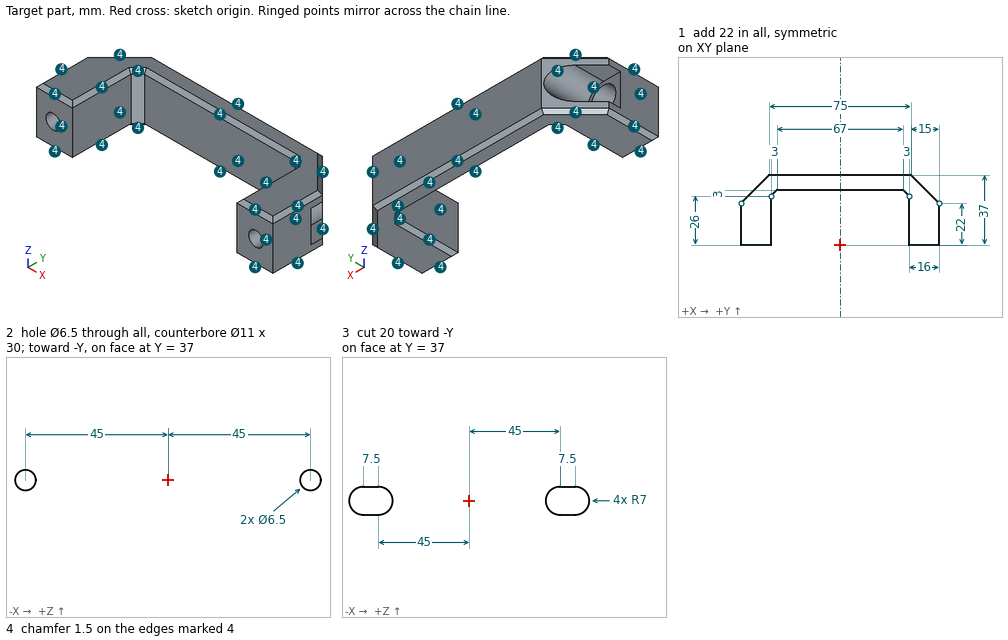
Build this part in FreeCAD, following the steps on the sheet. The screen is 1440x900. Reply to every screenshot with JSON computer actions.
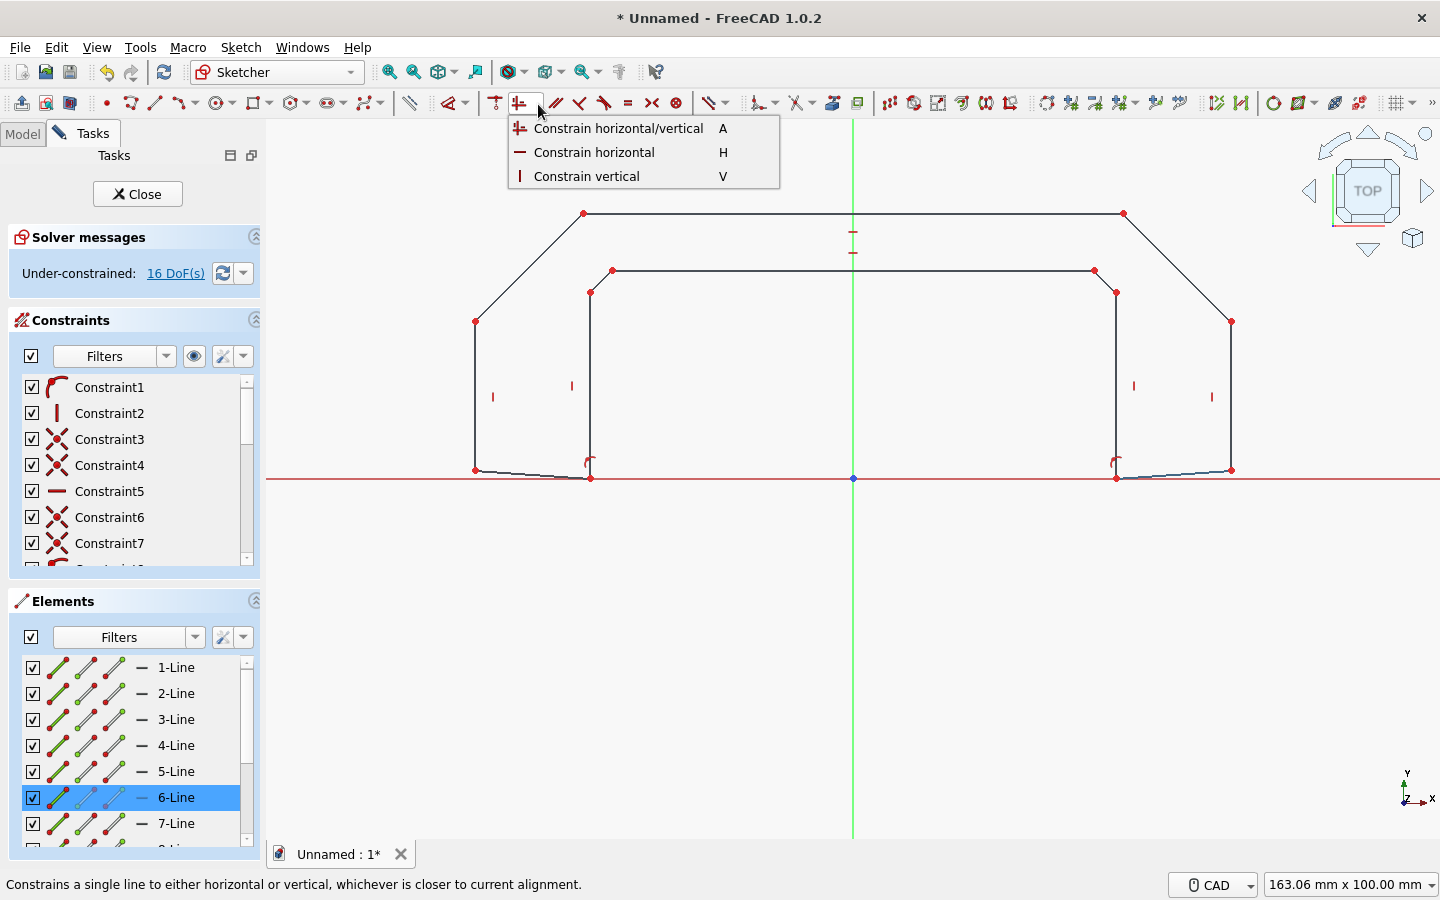
{"action": "left_click", "coordinate": [644, 152]}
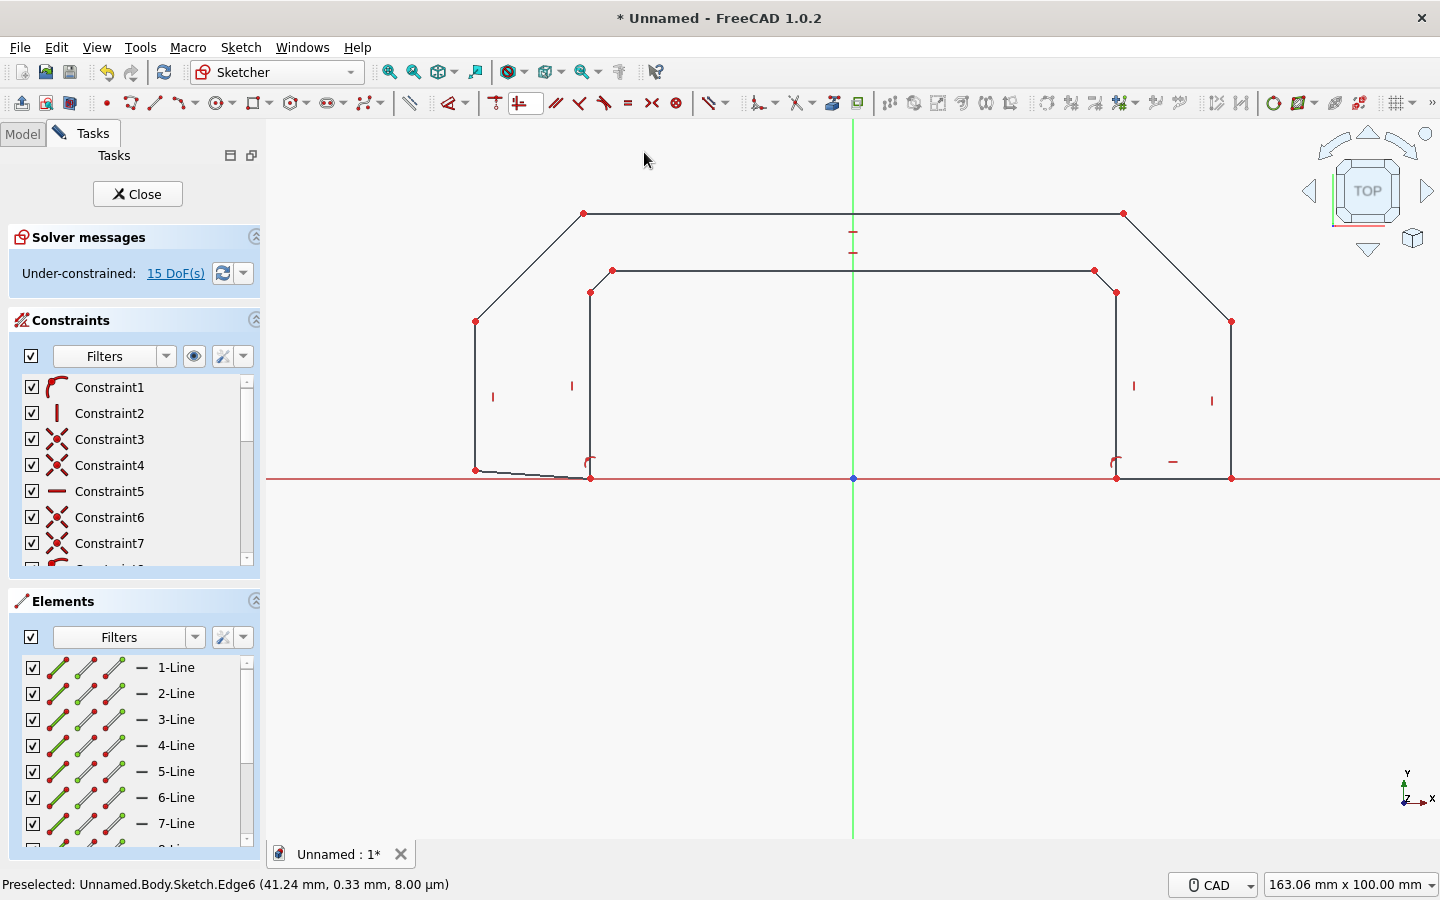
{"action": "left_click", "coordinate": [556, 477]}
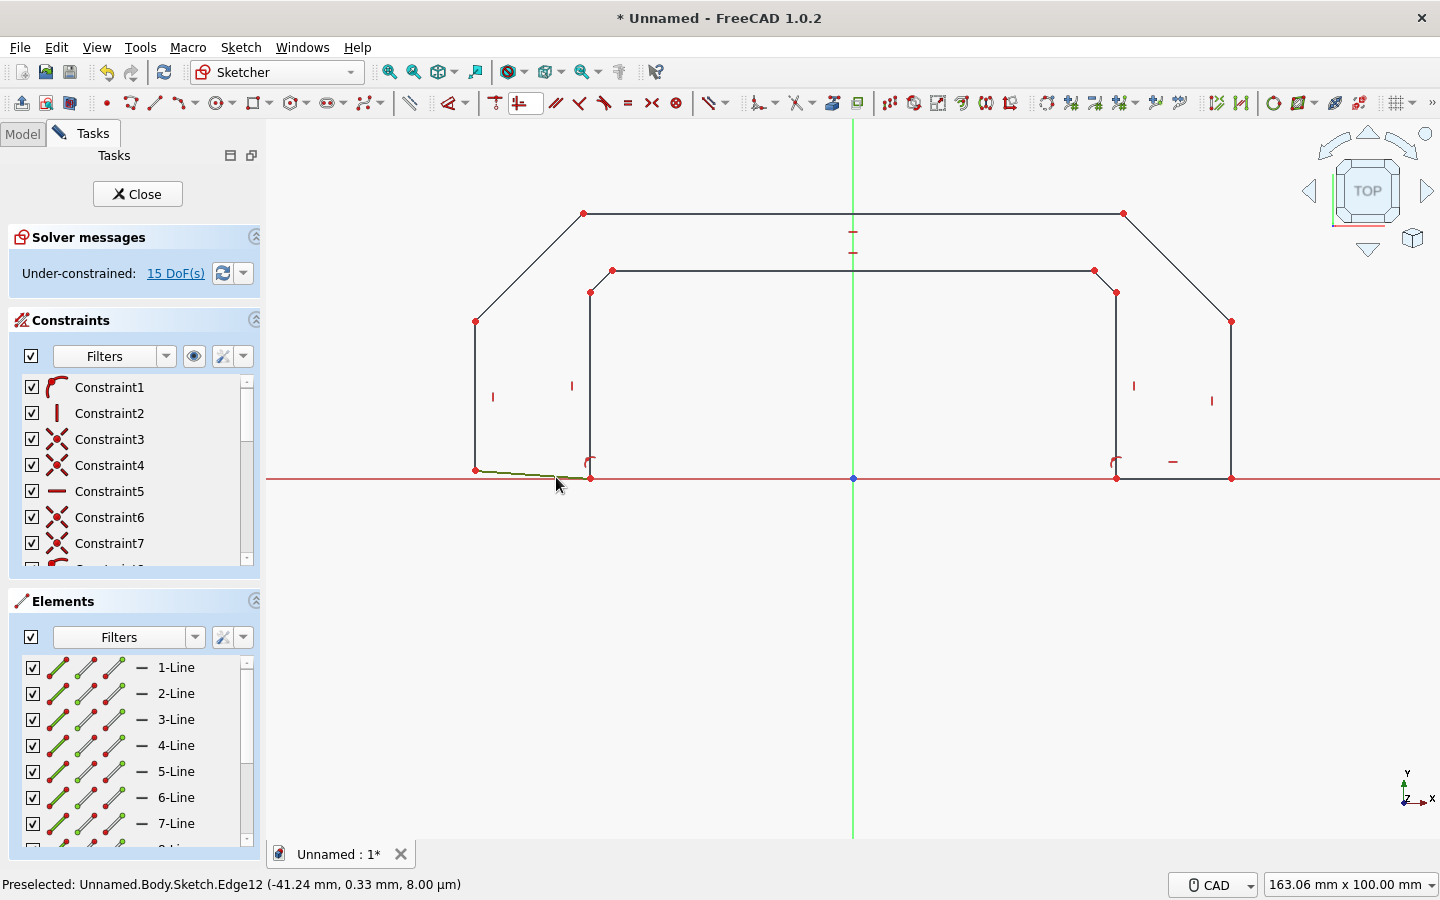
{"action": "key", "text": "h"}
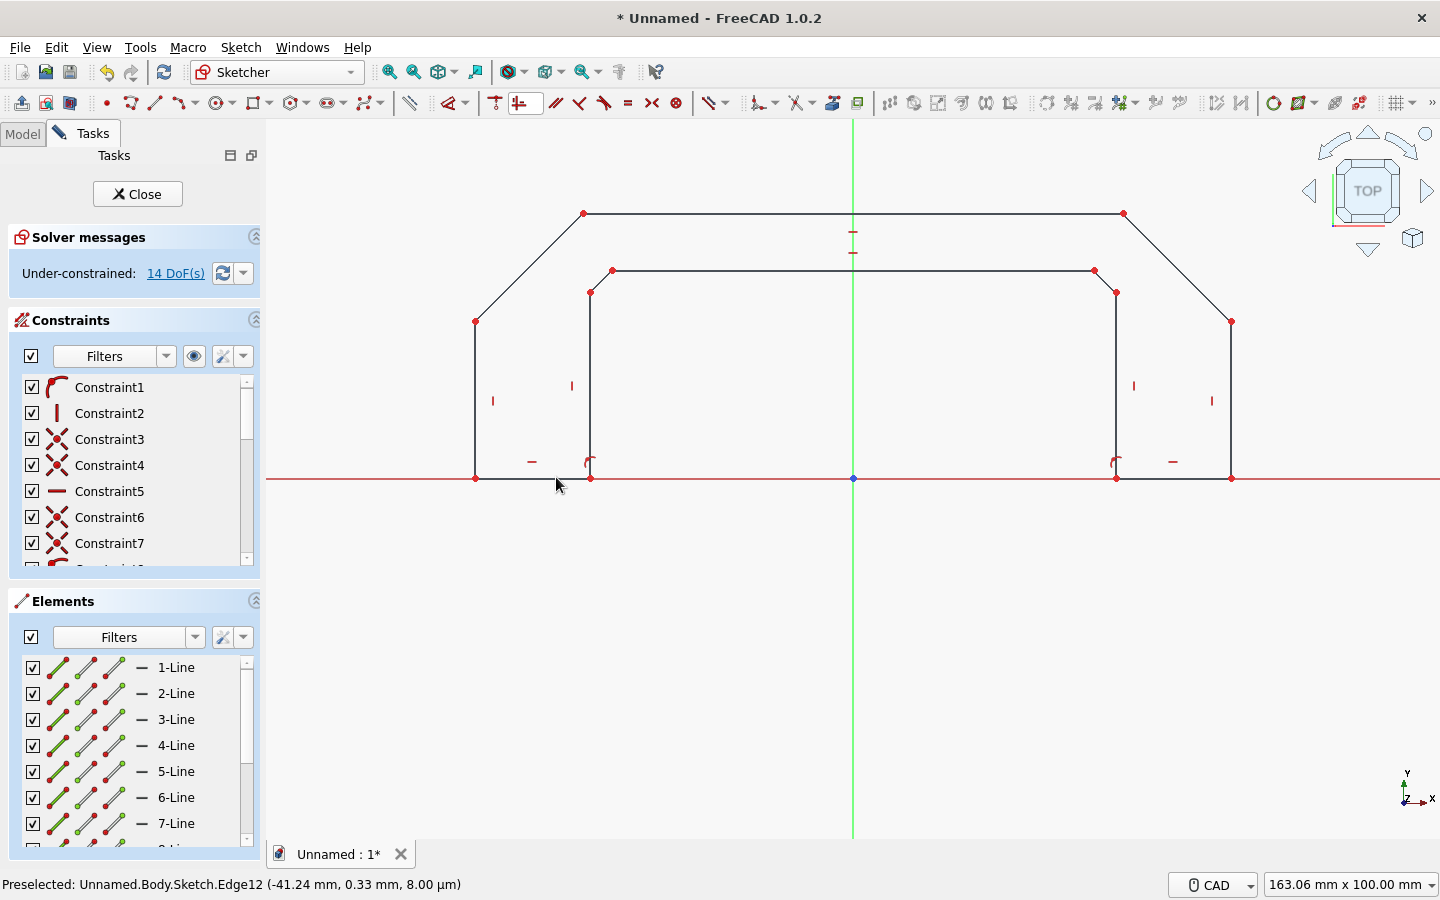
{"action": "left_click", "coordinate": [590, 293]}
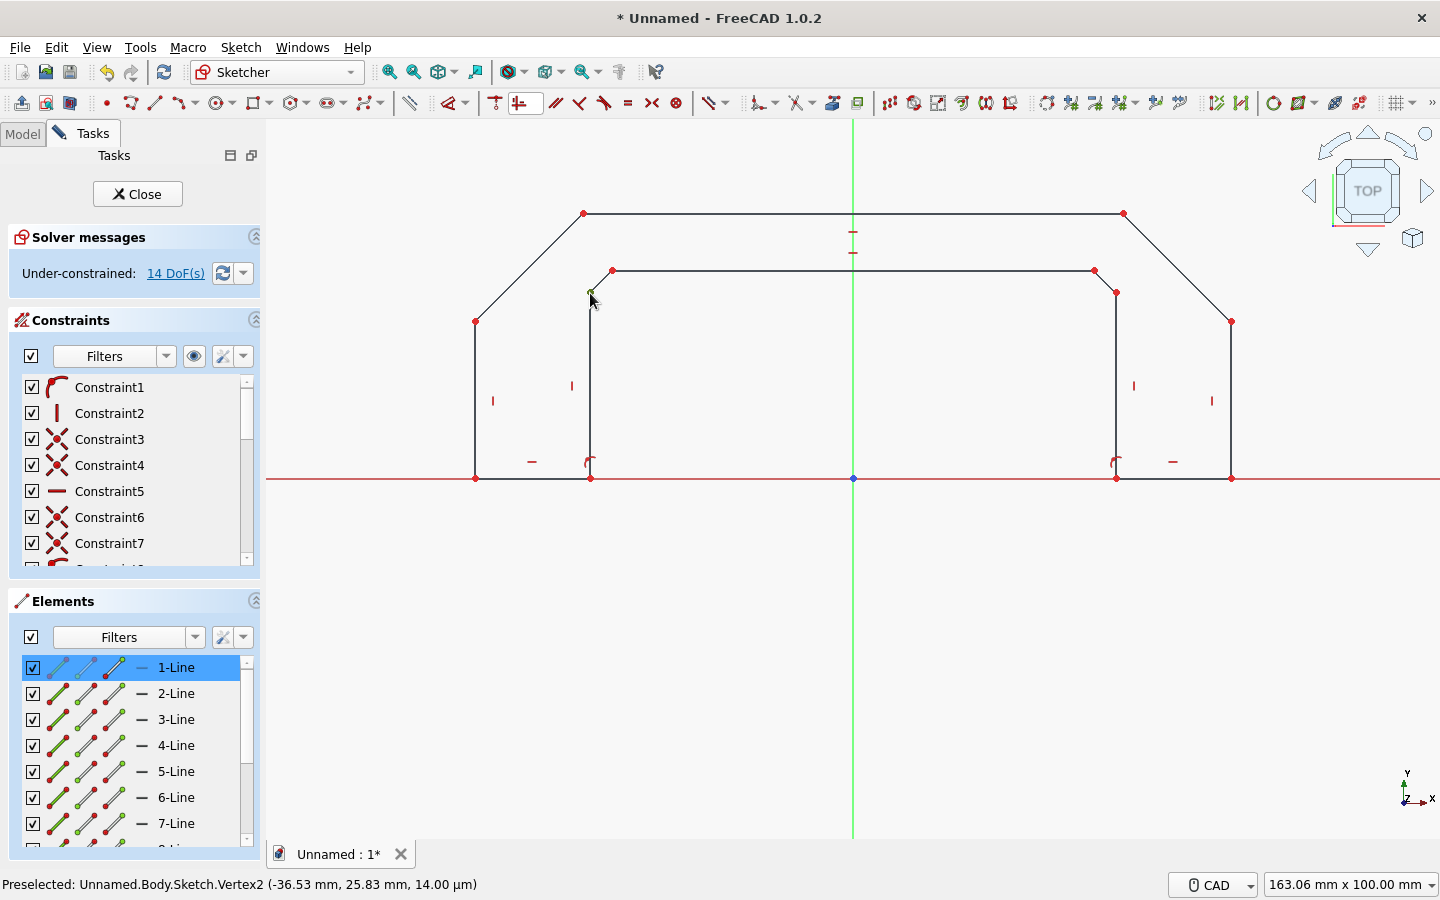
{"action": "left_click", "coordinate": [1116, 293]}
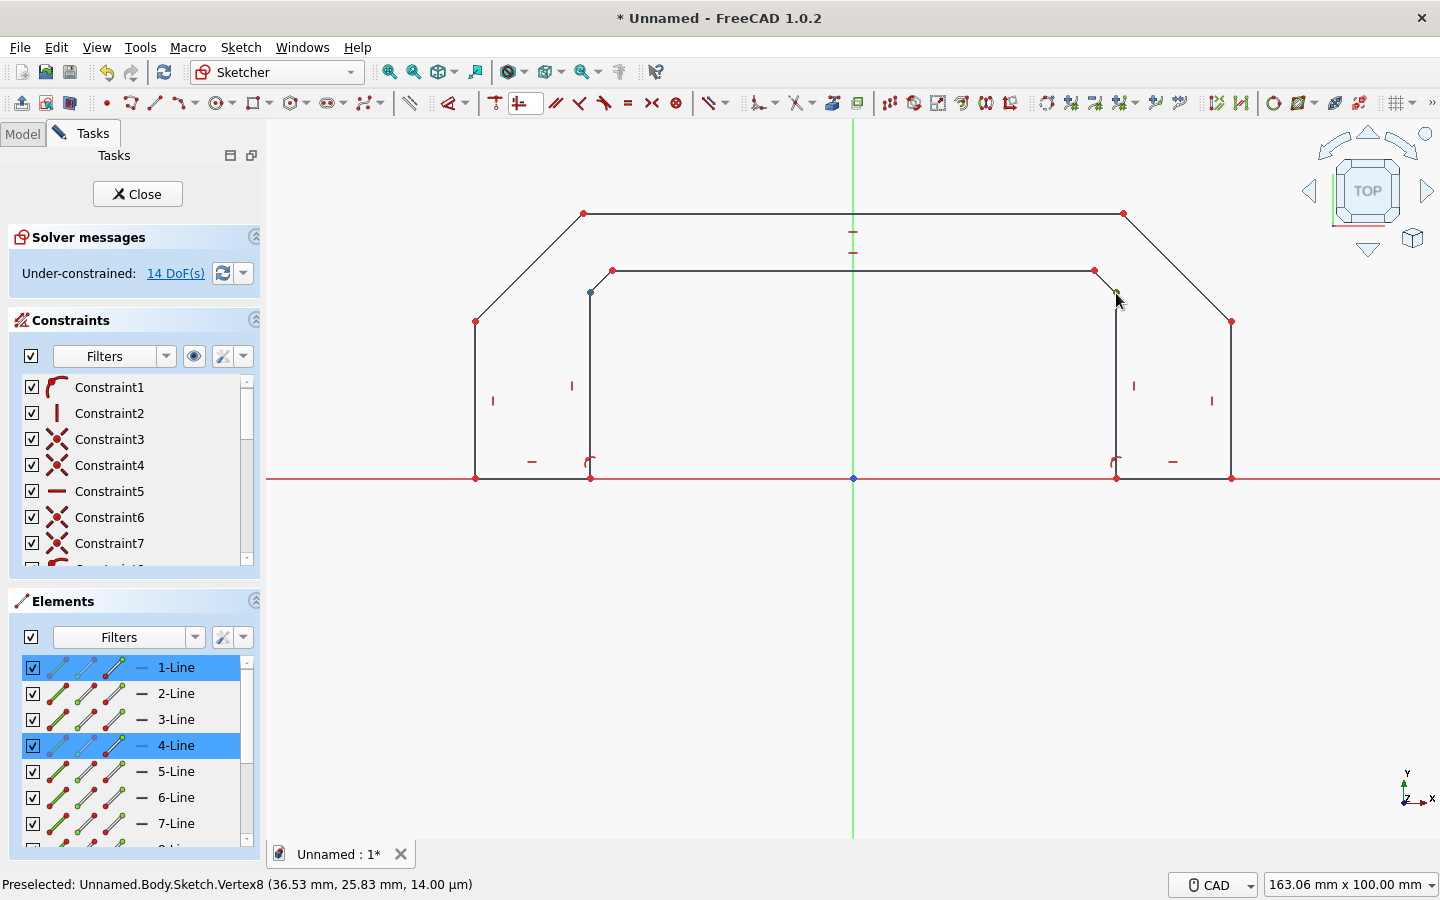
{"action": "left_click", "coordinate": [853, 764]}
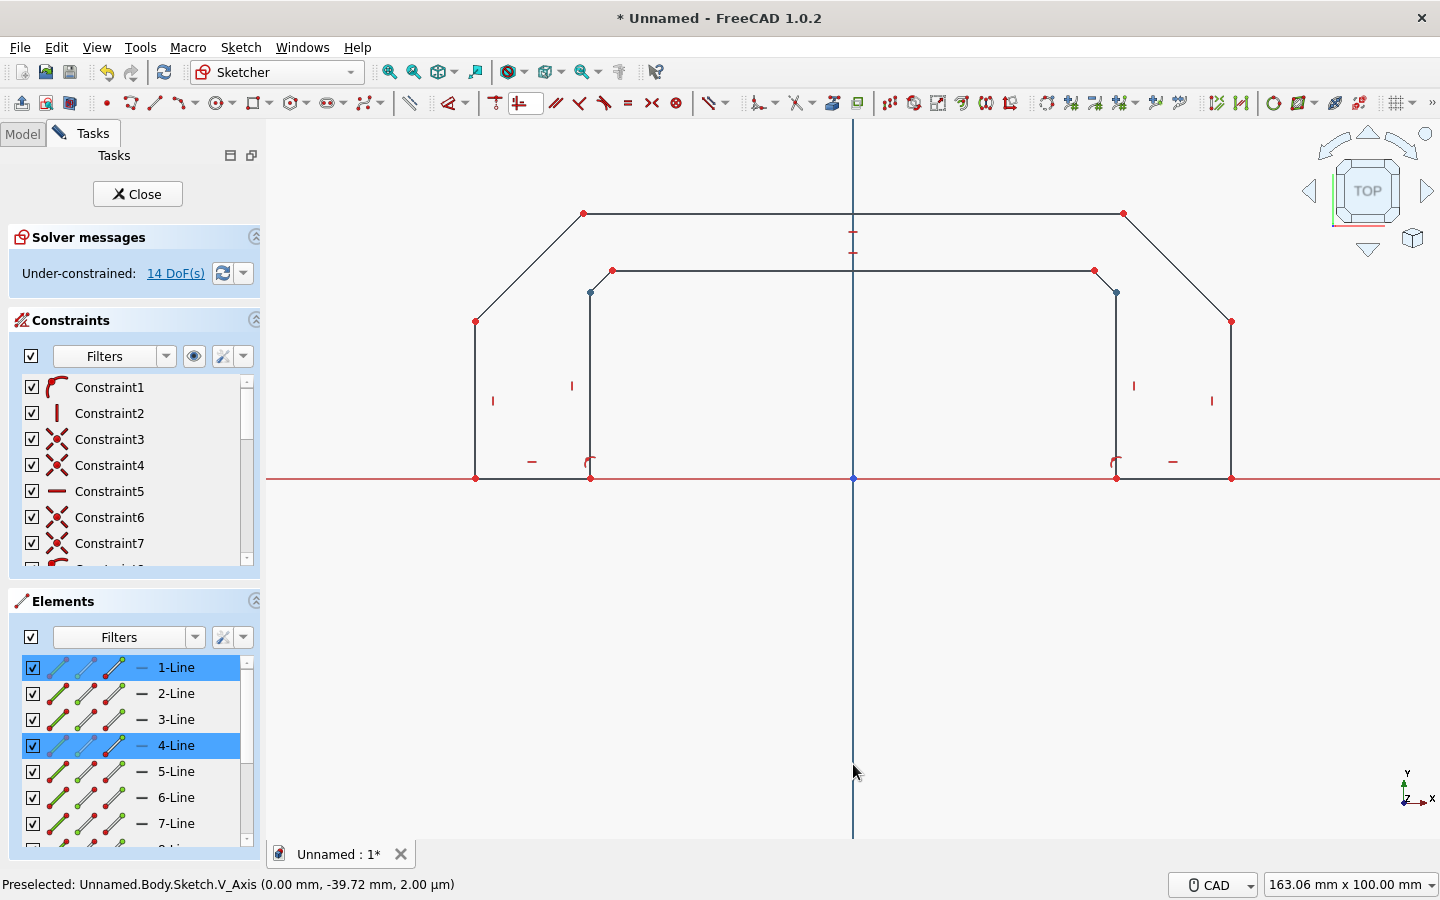
{"action": "left_click", "coordinate": [652, 104]}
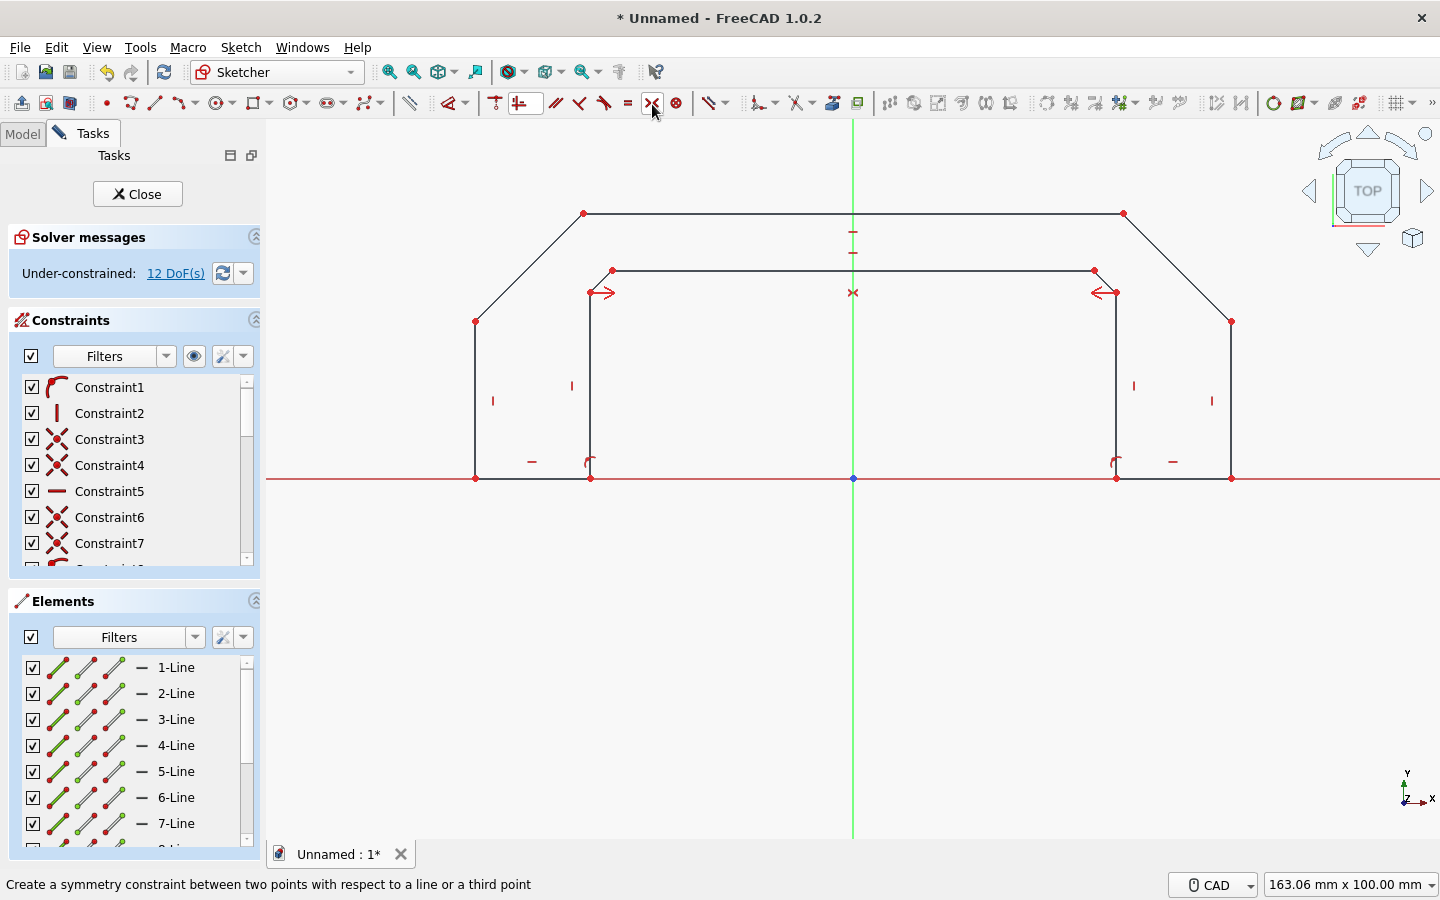
{"action": "left_click", "coordinate": [1231, 322]}